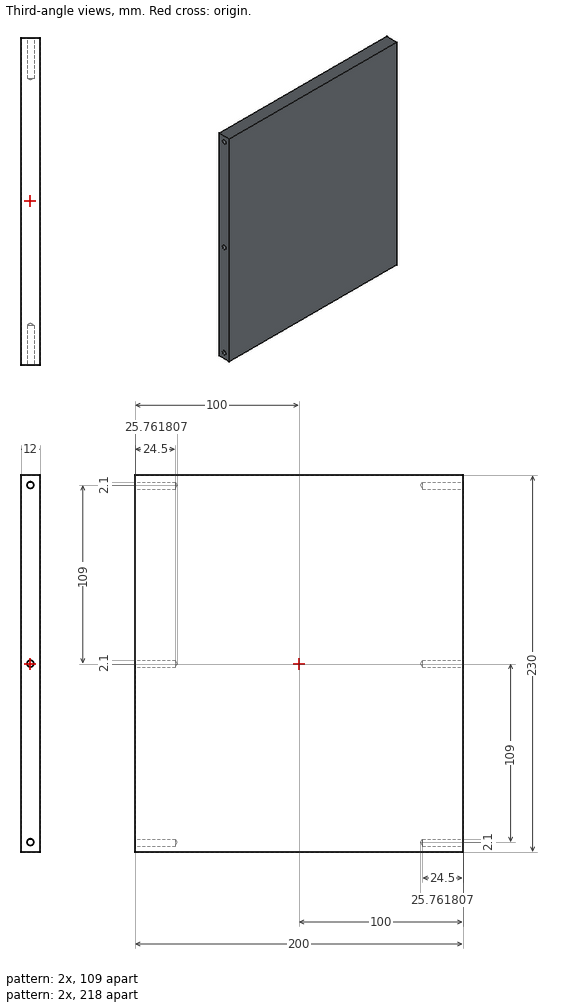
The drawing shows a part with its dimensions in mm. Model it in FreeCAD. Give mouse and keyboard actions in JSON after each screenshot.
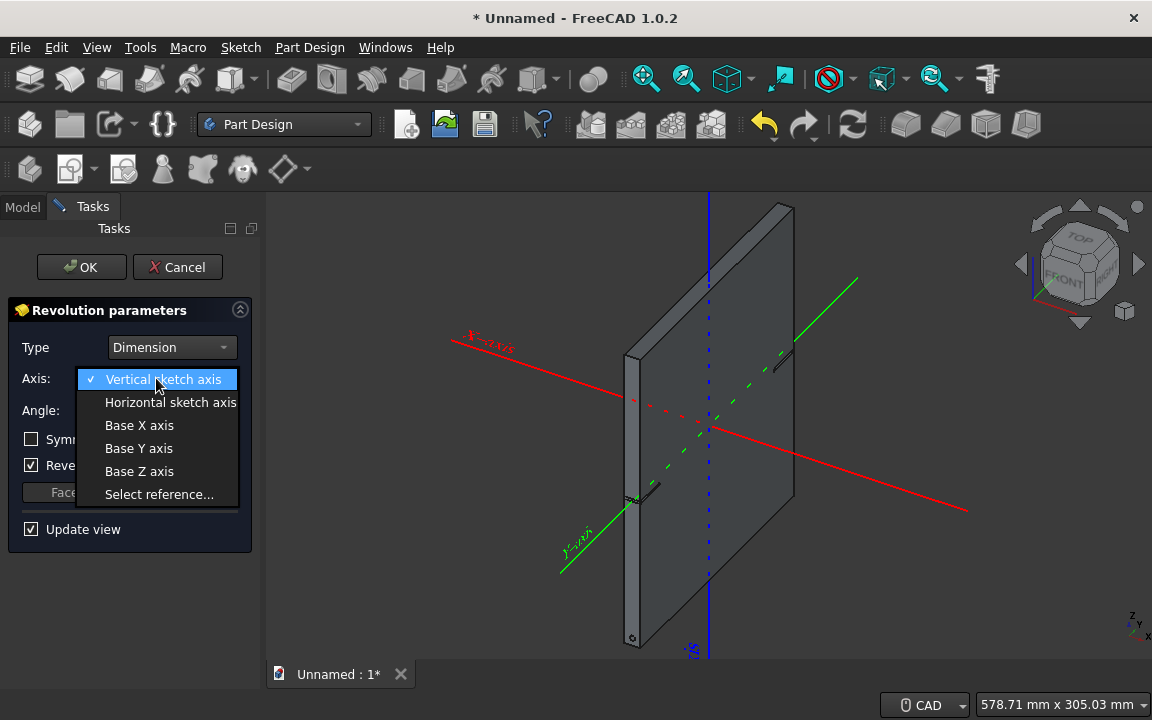
{"action": "left_click", "coordinate": [156, 402]}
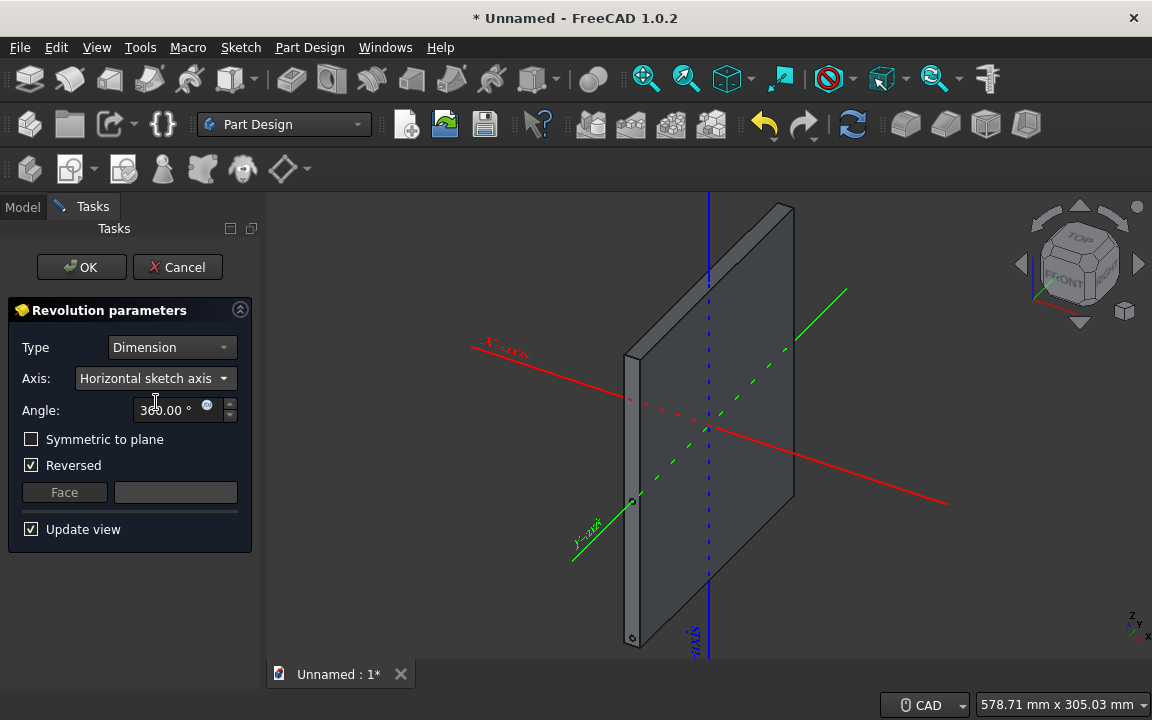
{"action": "left_click", "coordinate": [82, 267]}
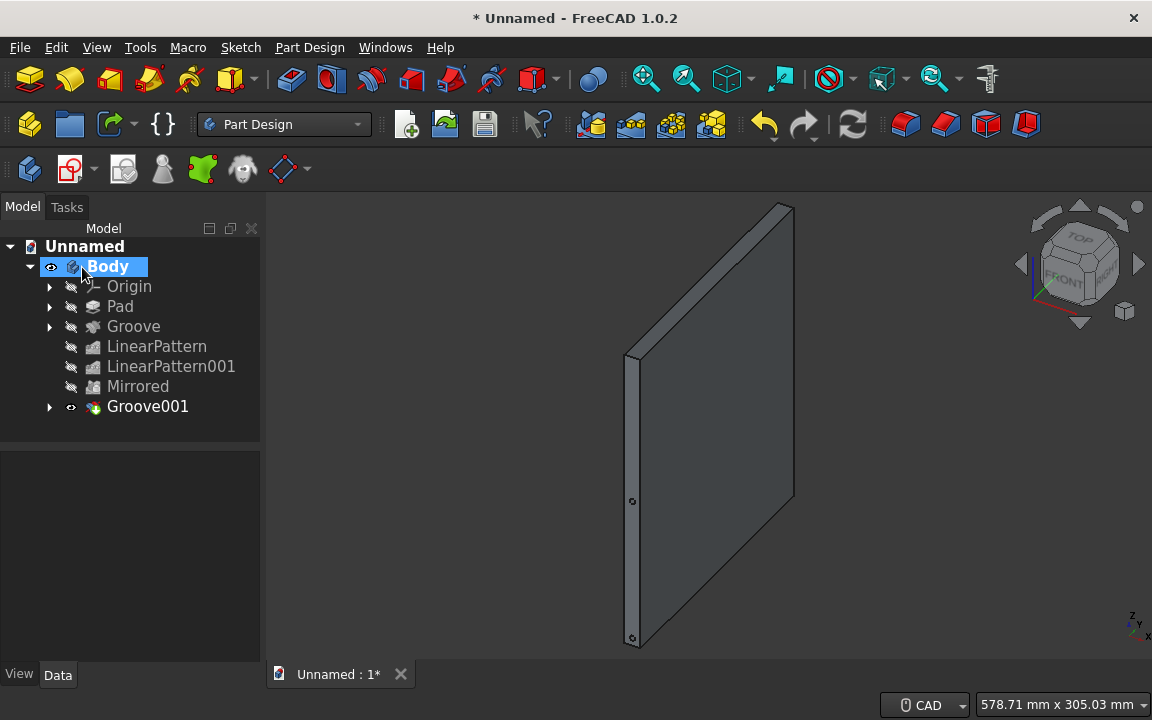
{"action": "left_click", "coordinate": [70, 170]}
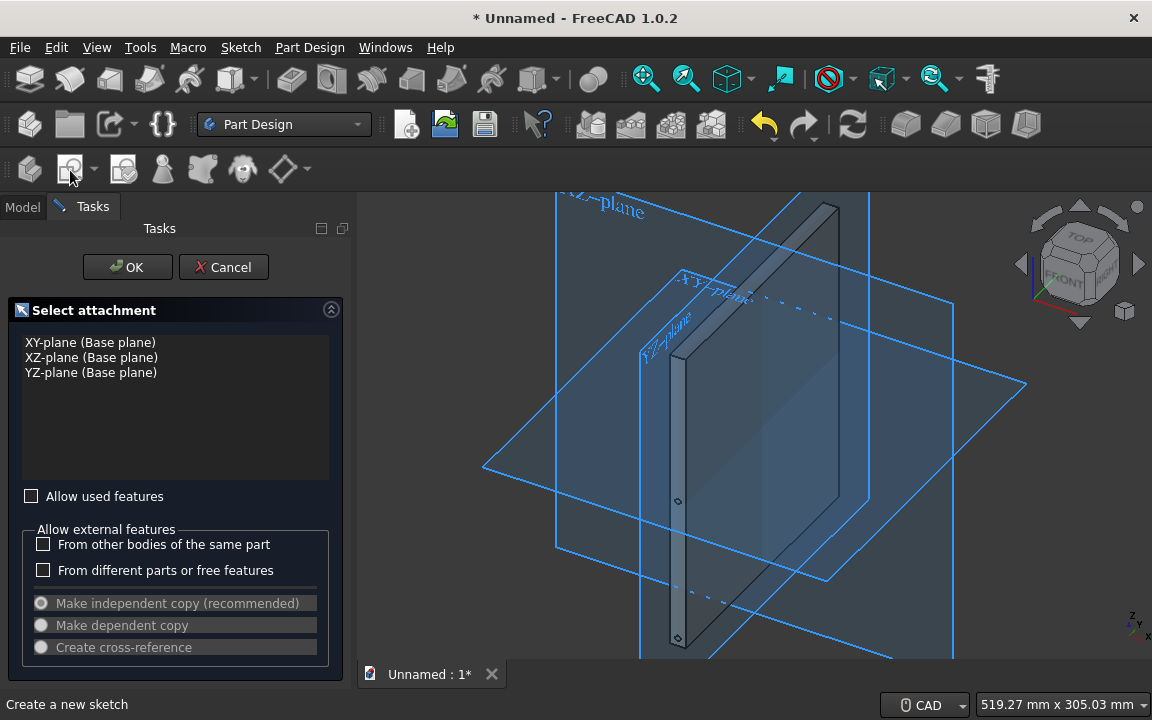
{"action": "left_click", "coordinate": [82, 372]}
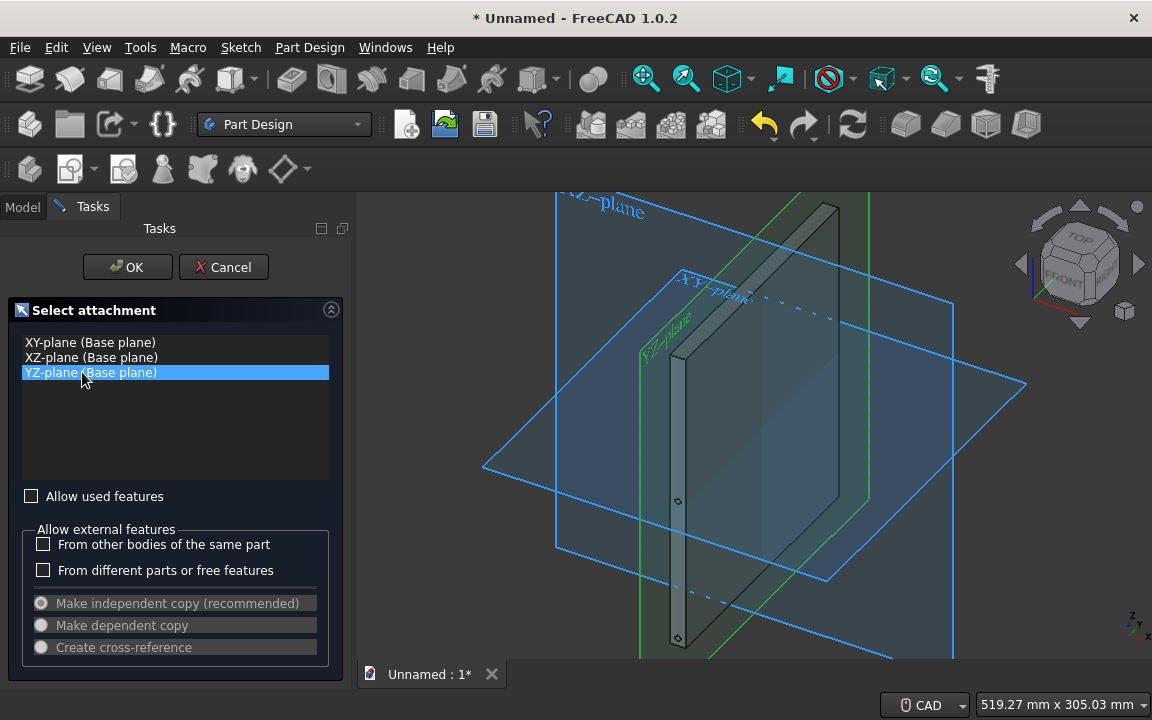
{"action": "left_click", "coordinate": [128, 267]}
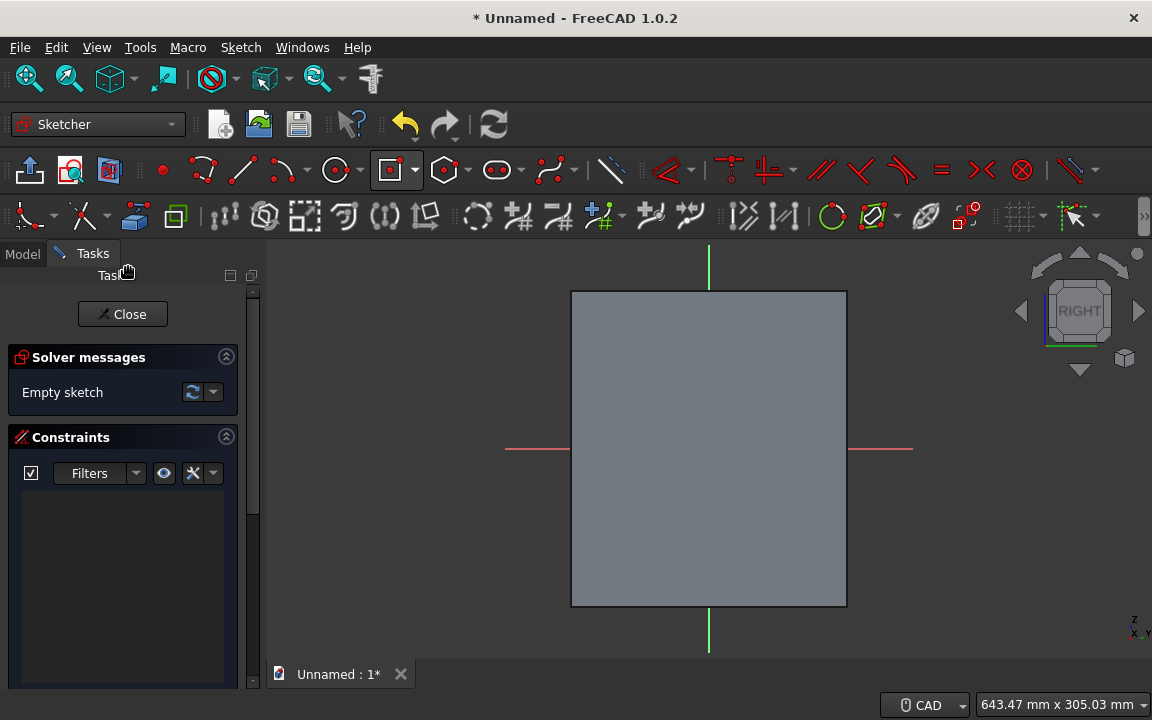
{"action": "left_click", "coordinate": [110, 170]}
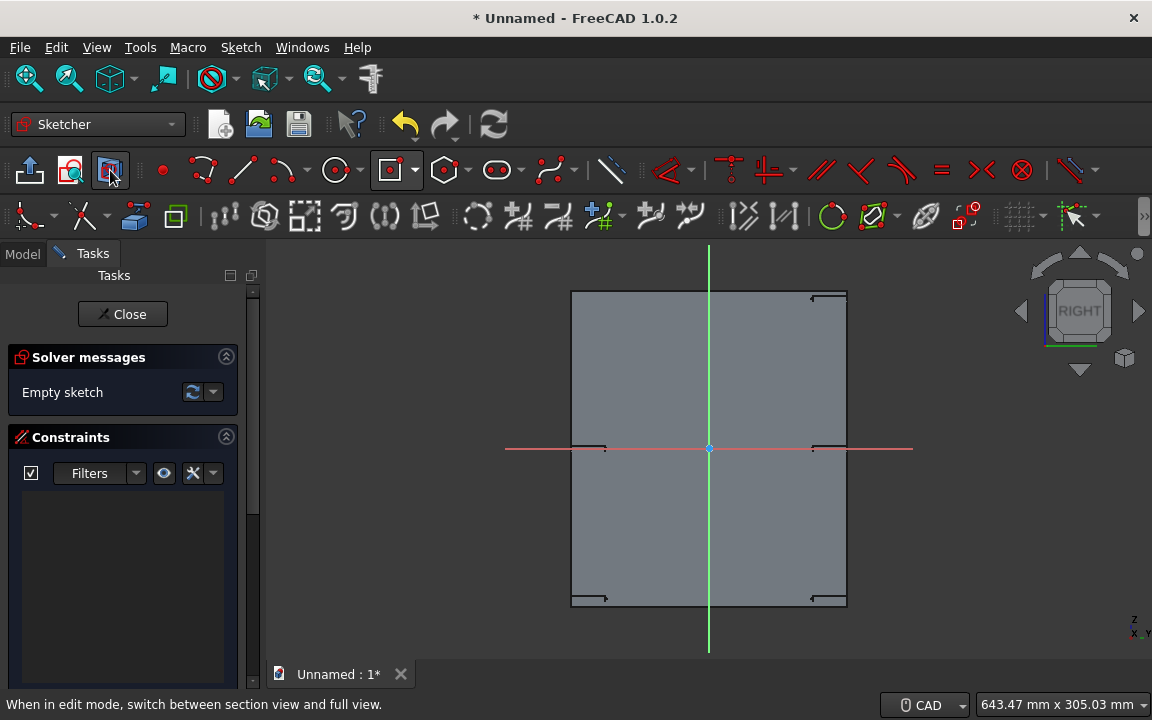
{"action": "scroll", "coordinate": [575, 279], "scroll_direction": "up", "scroll_amount": 11}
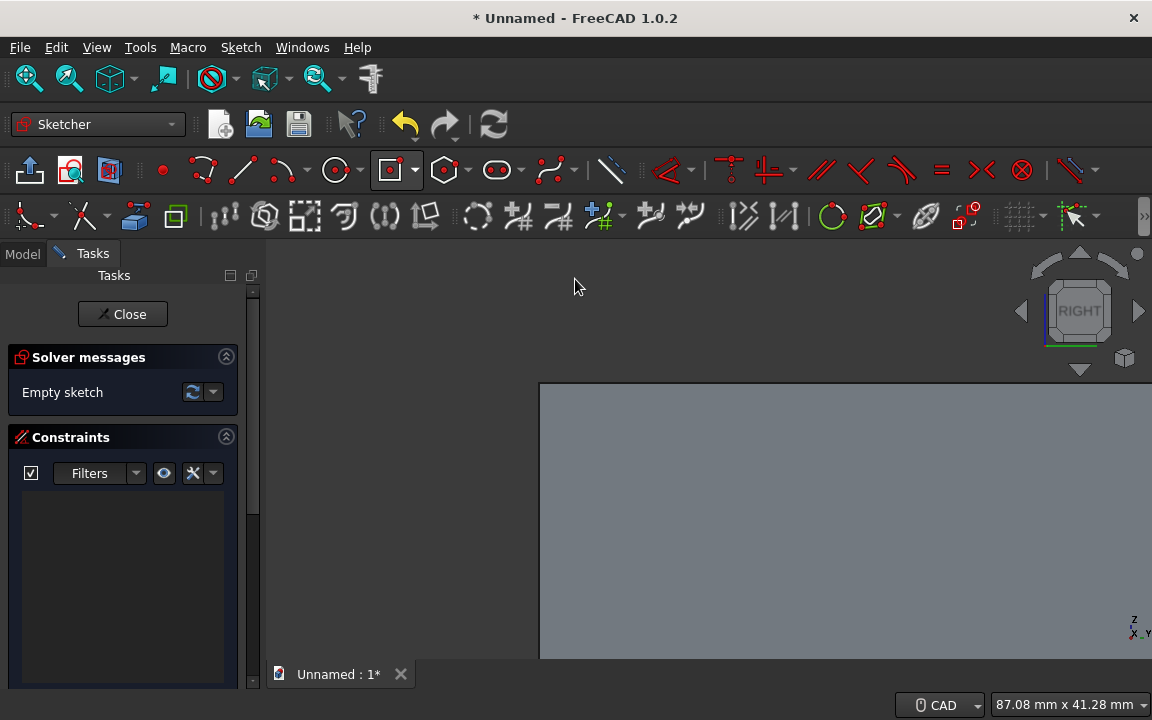
{"action": "left_click", "coordinate": [204, 170]}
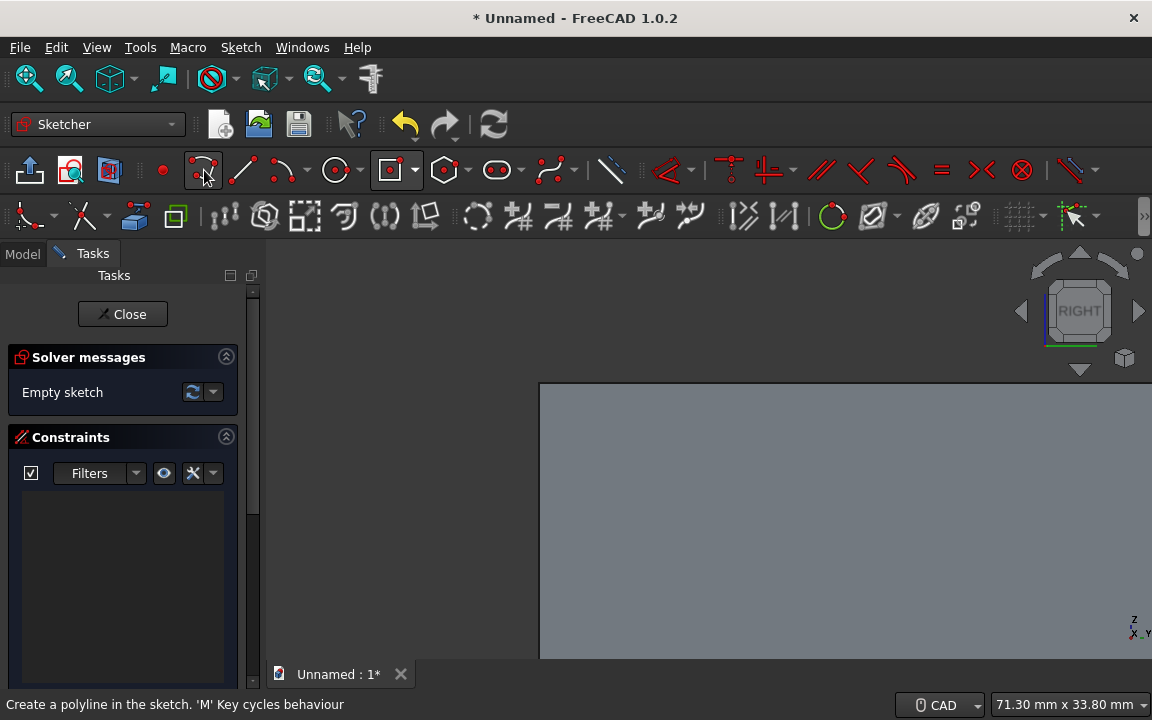
{"action": "left_click", "coordinate": [859, 458]}
{"action": "left_click", "coordinate": [843, 432]}
{"action": "left_click", "coordinate": [539, 432]}
{"action": "left_click", "coordinate": [539, 458]}
{"action": "left_click", "coordinate": [859, 459]}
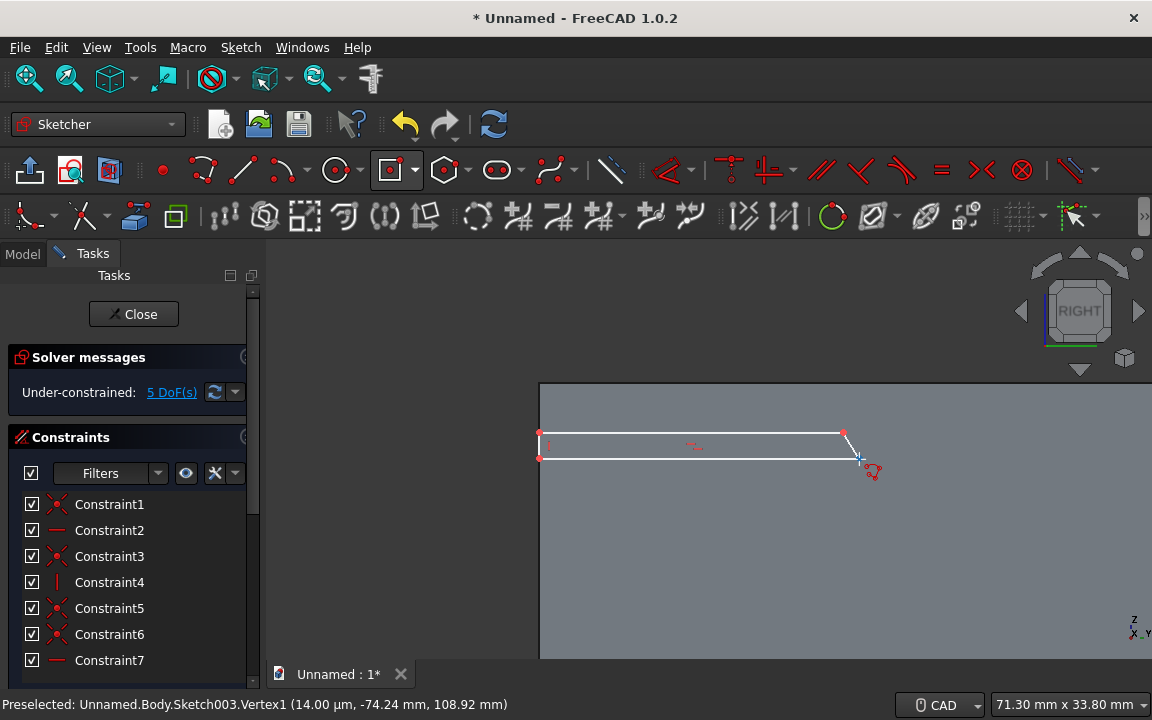
{"action": "left_click", "coordinate": [244, 170]}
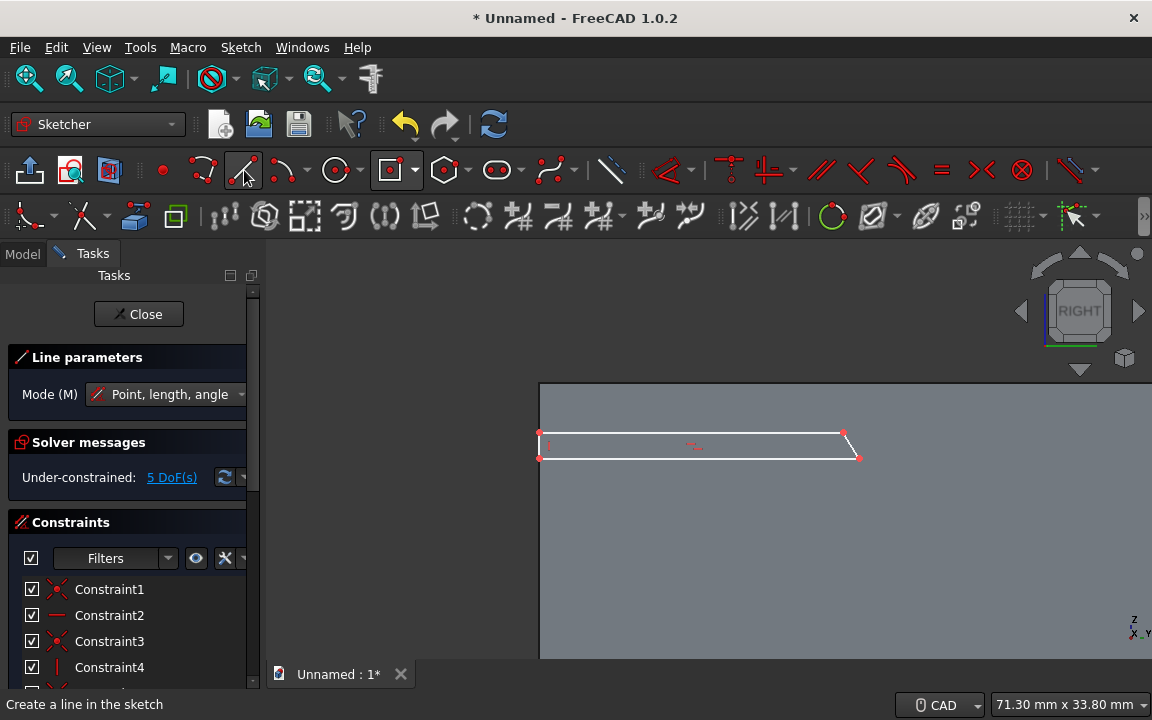
{"action": "left_click", "coordinate": [507, 458]}
{"action": "left_click", "coordinate": [411, 458]}
{"action": "key", "text": "Escape"}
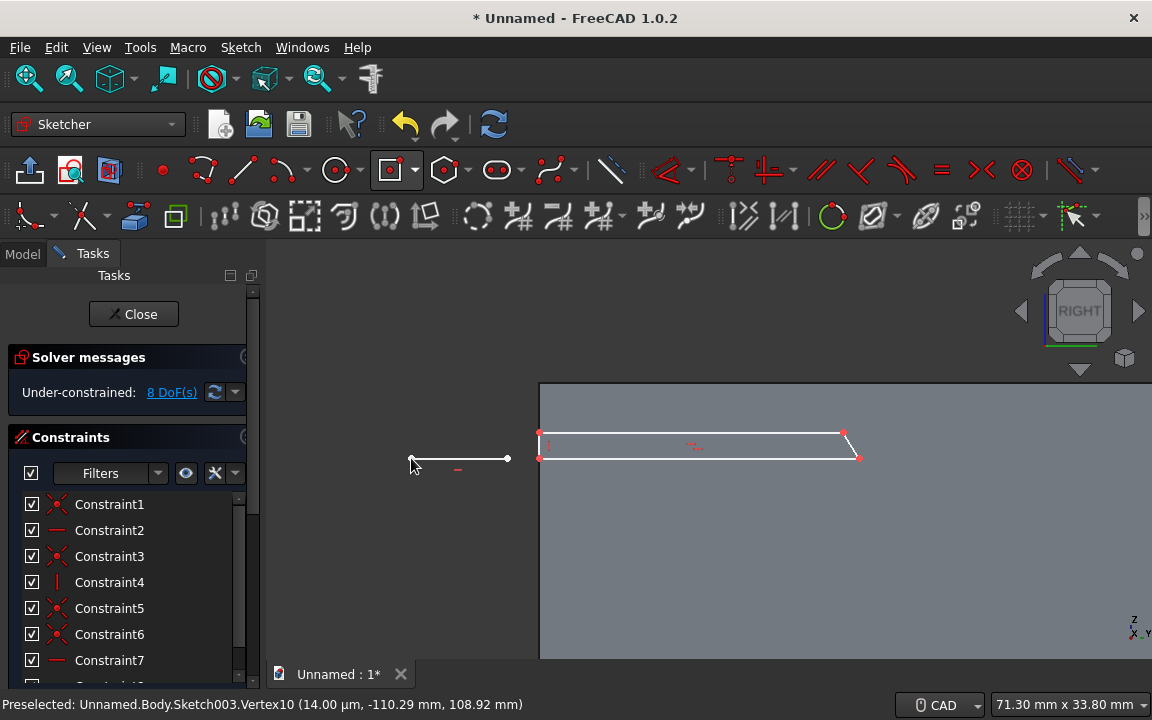
{"action": "left_click", "coordinate": [478, 459]}